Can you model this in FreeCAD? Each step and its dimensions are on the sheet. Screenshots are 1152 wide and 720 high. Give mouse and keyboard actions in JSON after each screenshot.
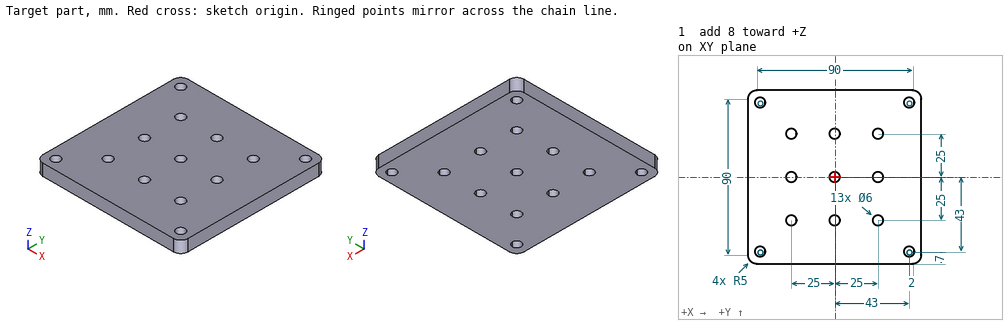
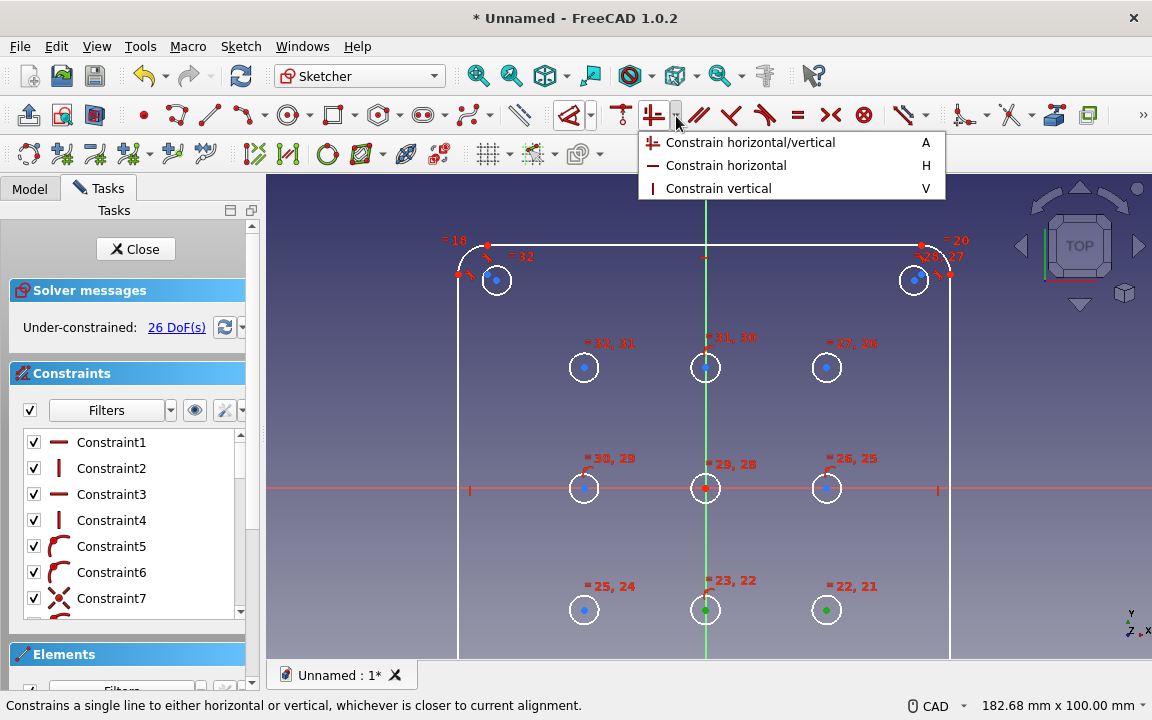
{"action": "left_click", "coordinate": [792, 166]}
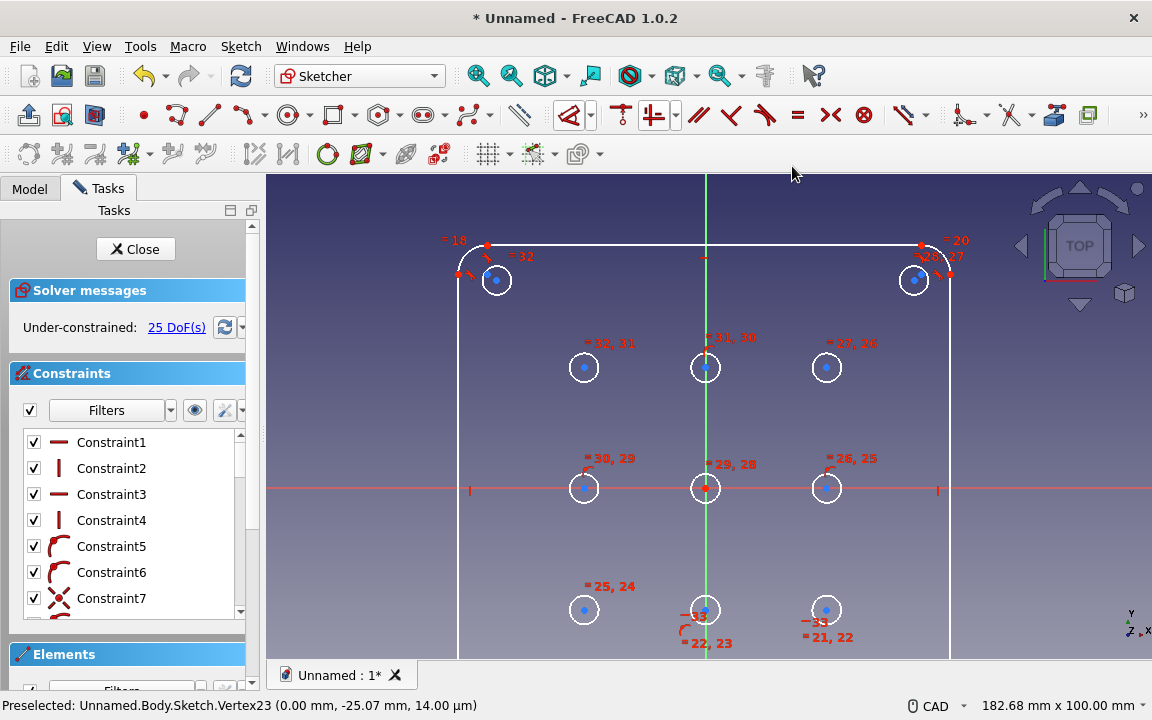
{"action": "scroll", "coordinate": [706, 610], "scroll_direction": "up", "scroll_amount": 4}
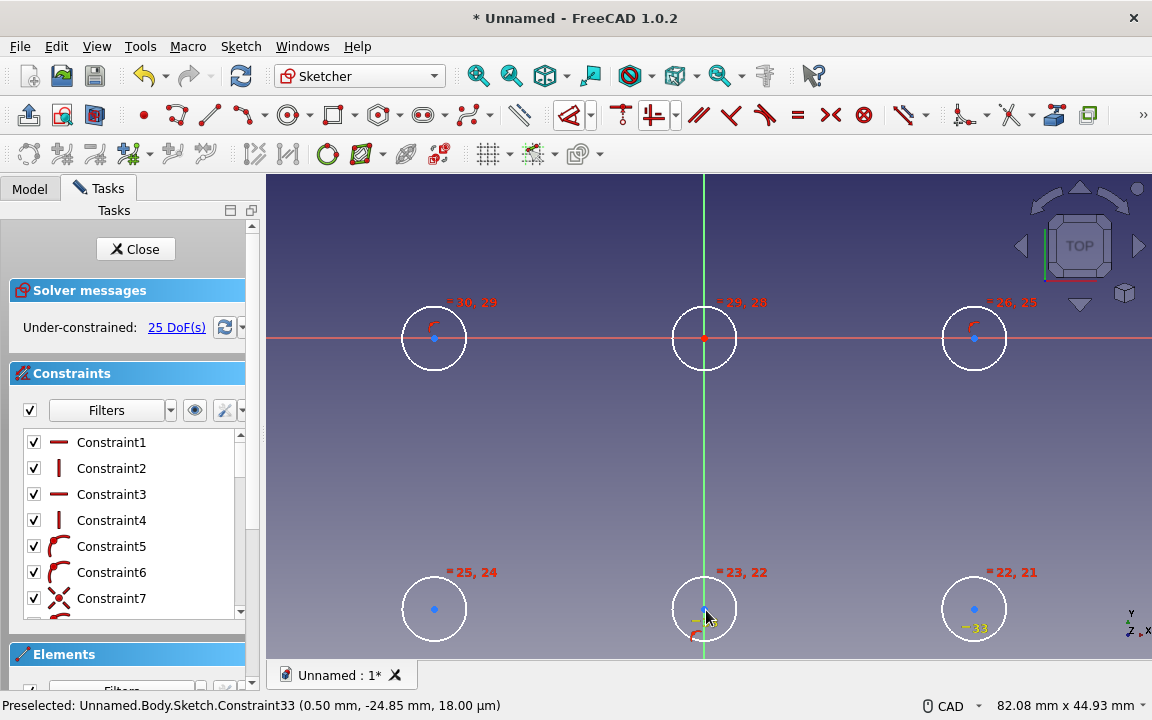
{"action": "left_click", "coordinate": [704, 609]}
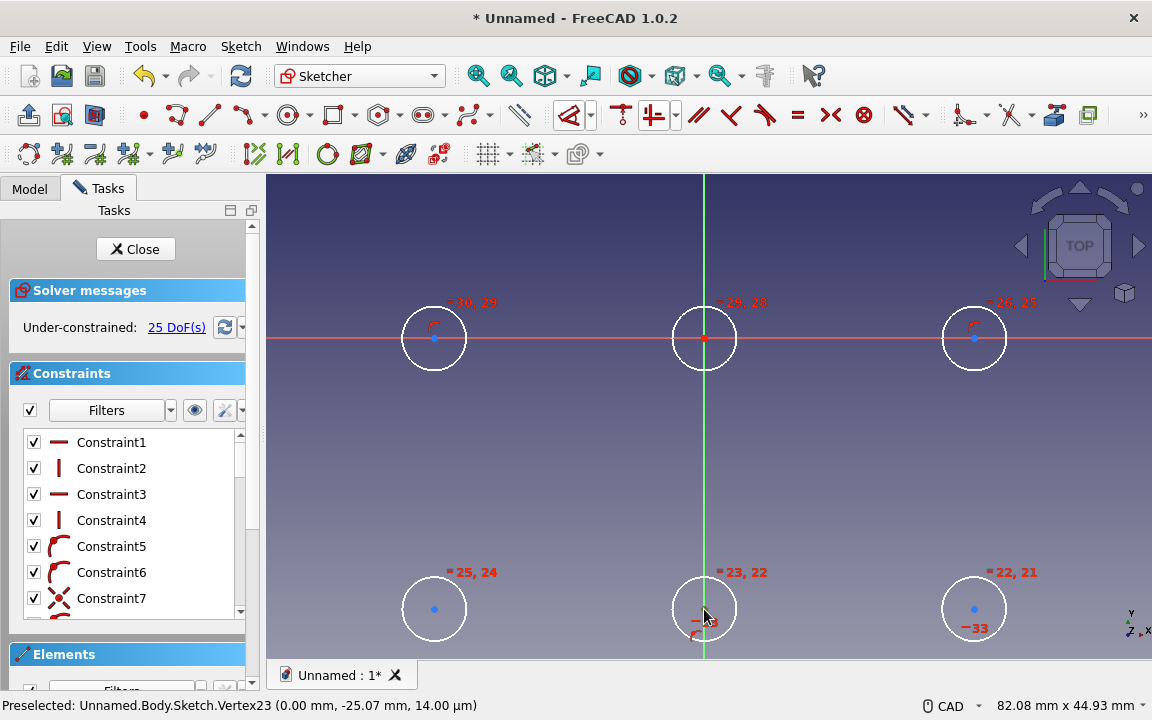
{"action": "left_click", "coordinate": [434, 609]}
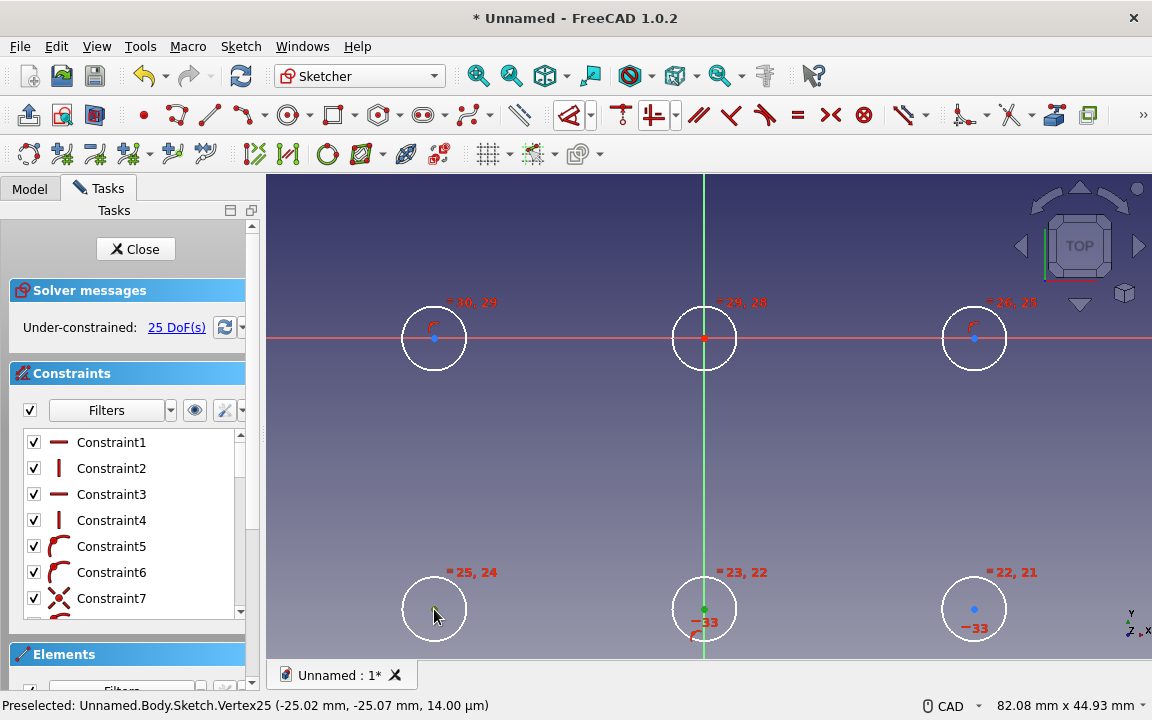
{"action": "key", "text": "h"}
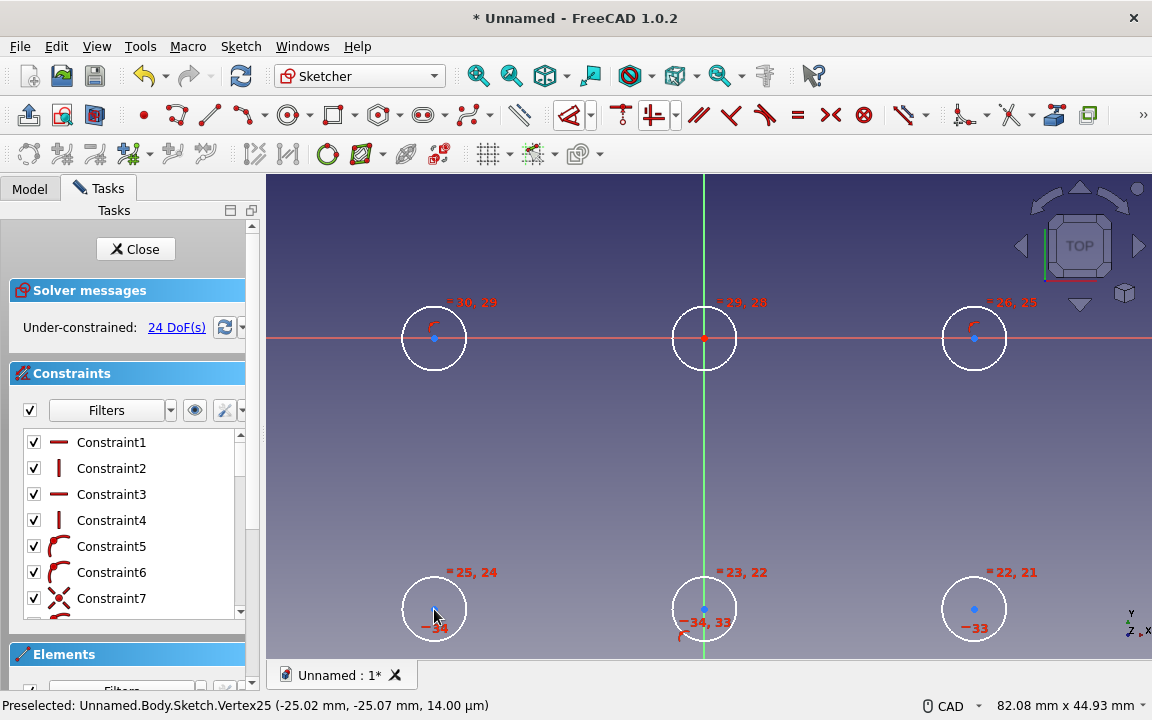
{"action": "left_click", "coordinate": [974, 609]}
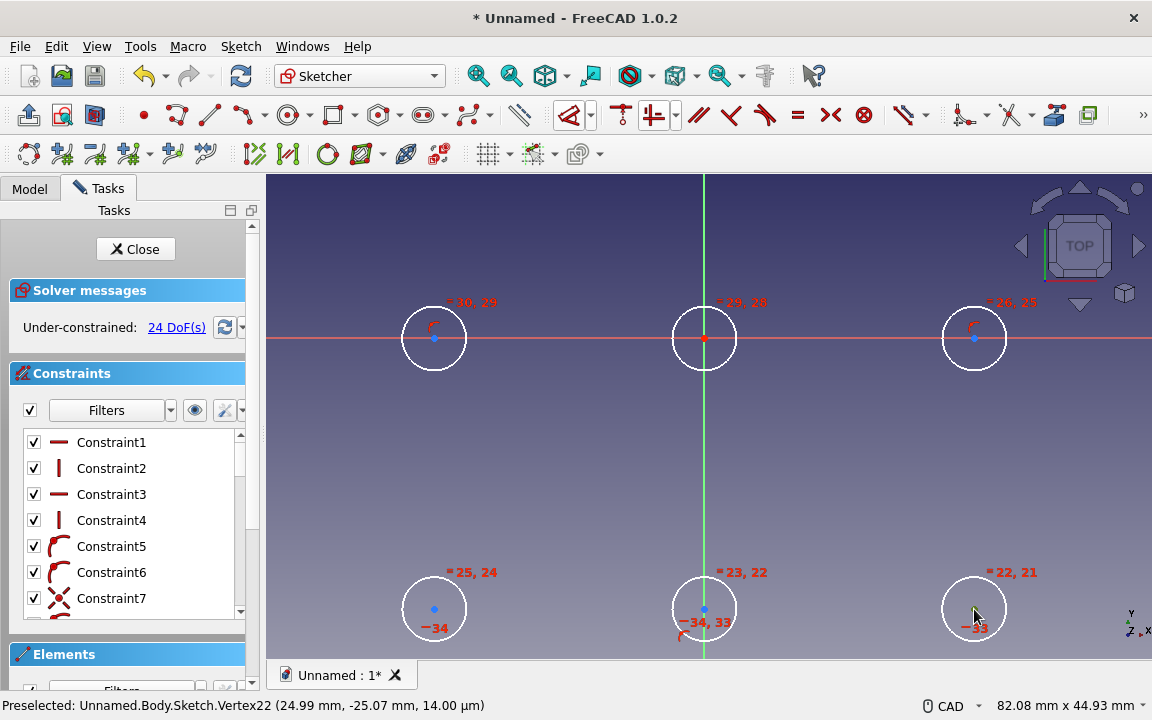
{"action": "left_click", "coordinate": [974, 338]}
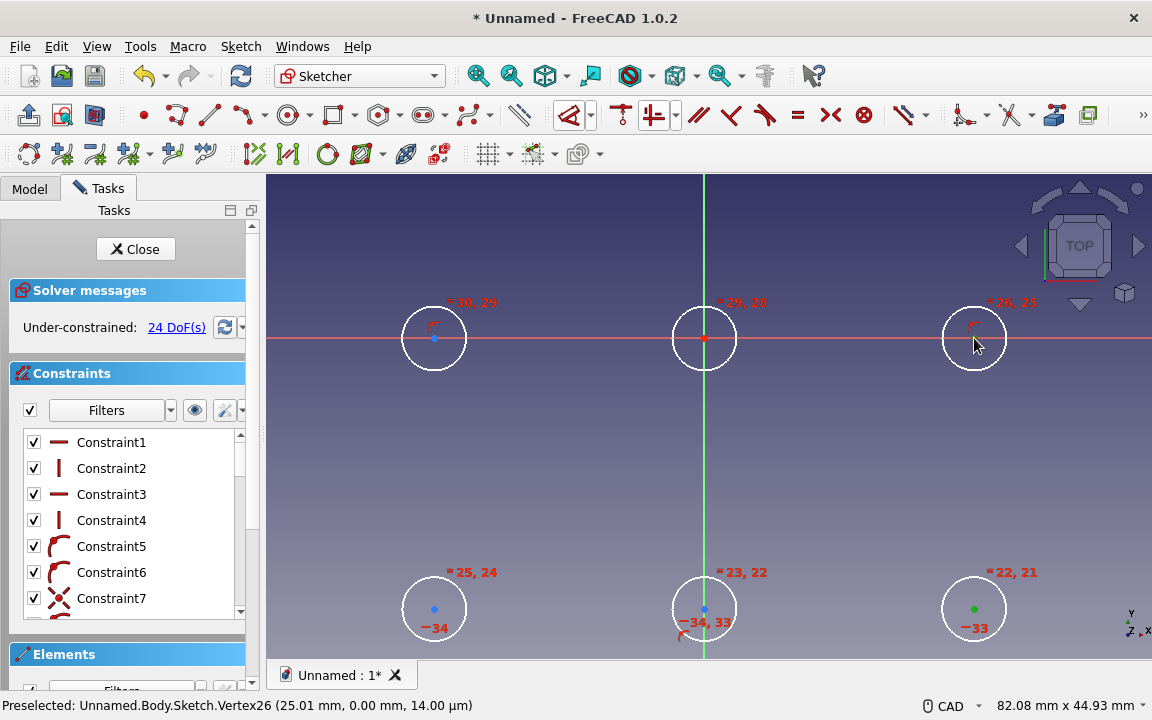
{"action": "key", "text": "v"}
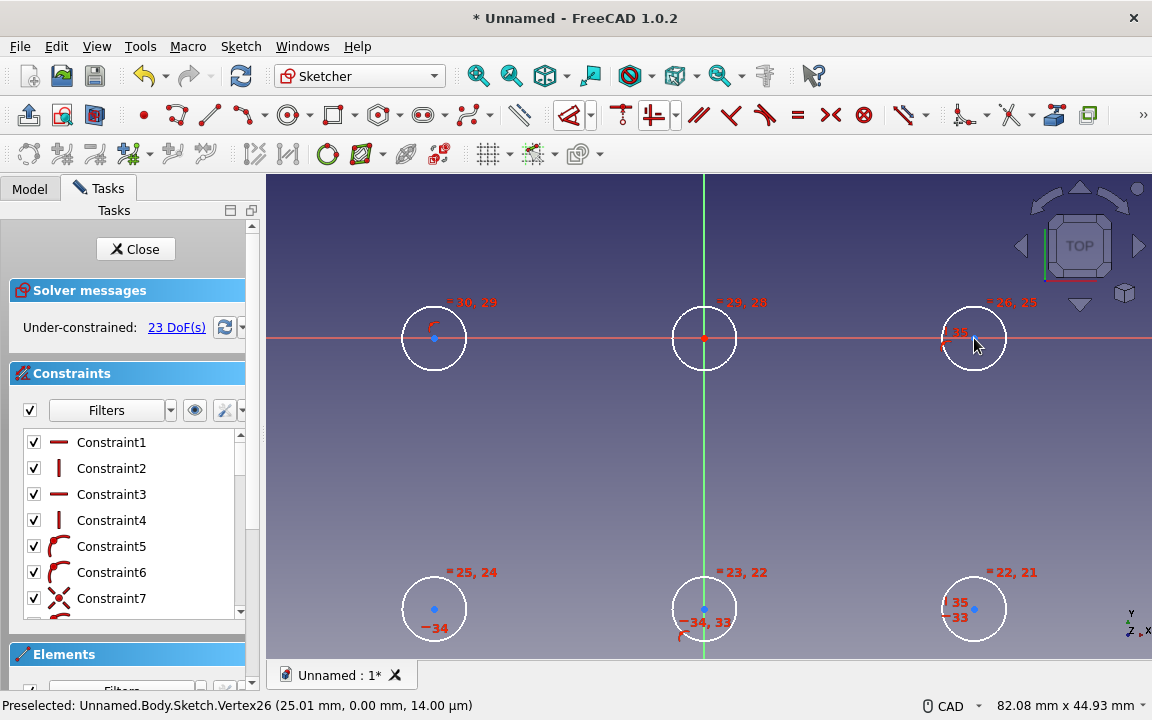
{"action": "left_click", "coordinate": [974, 338]}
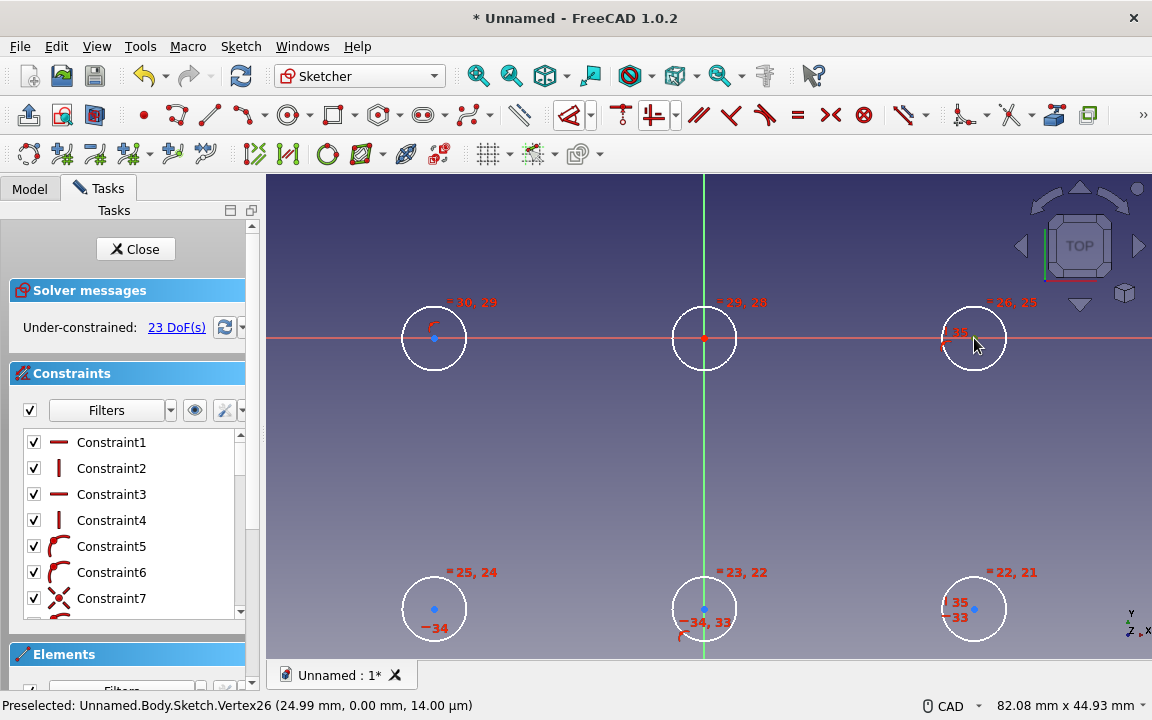
{"action": "scroll", "coordinate": [613, 450], "scroll_direction": "down", "scroll_amount": 6}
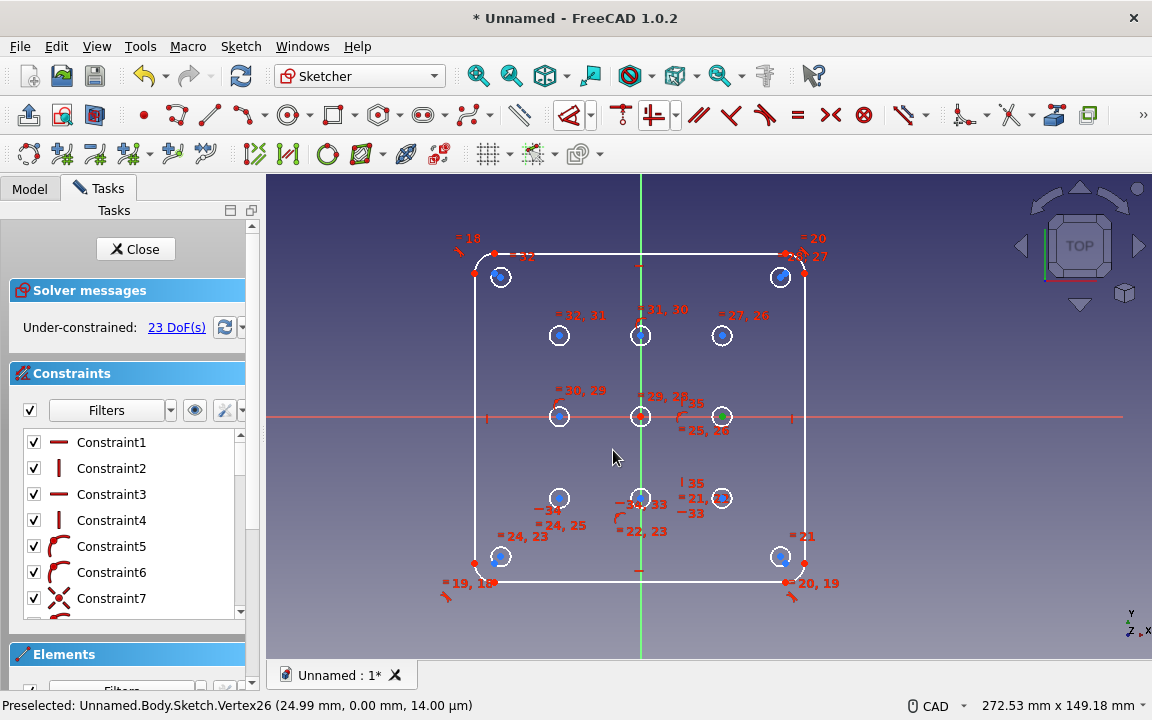
{"action": "left_click", "coordinate": [722, 336]}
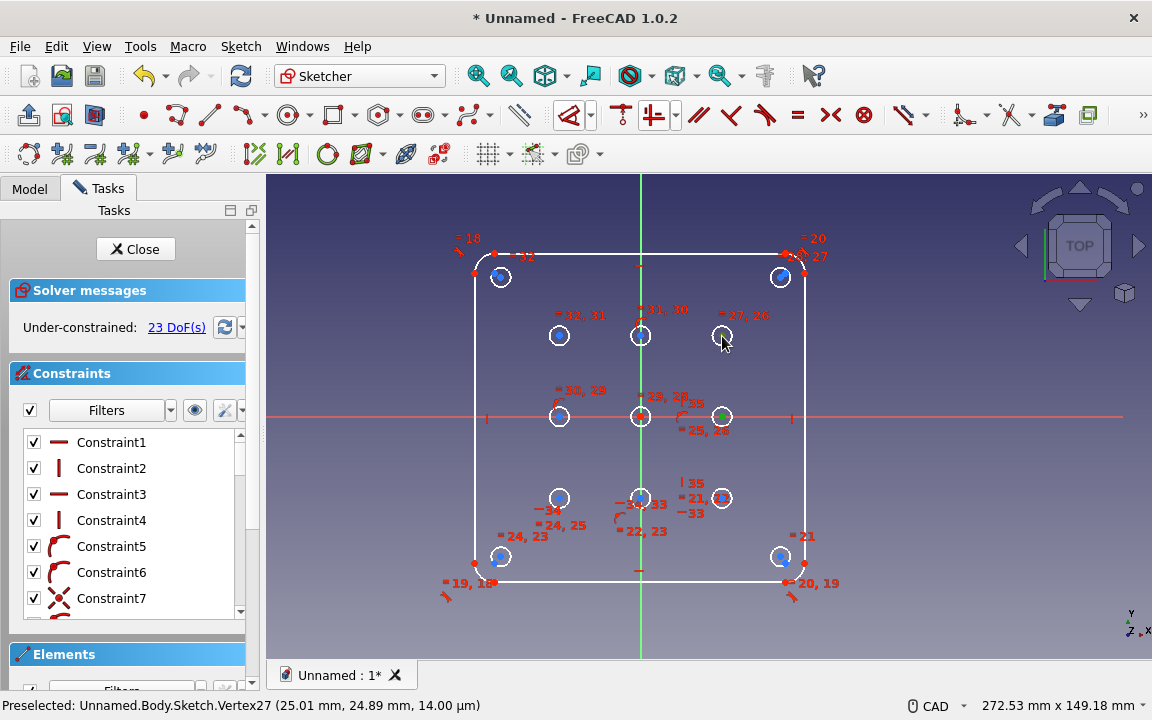
{"action": "key", "text": "v"}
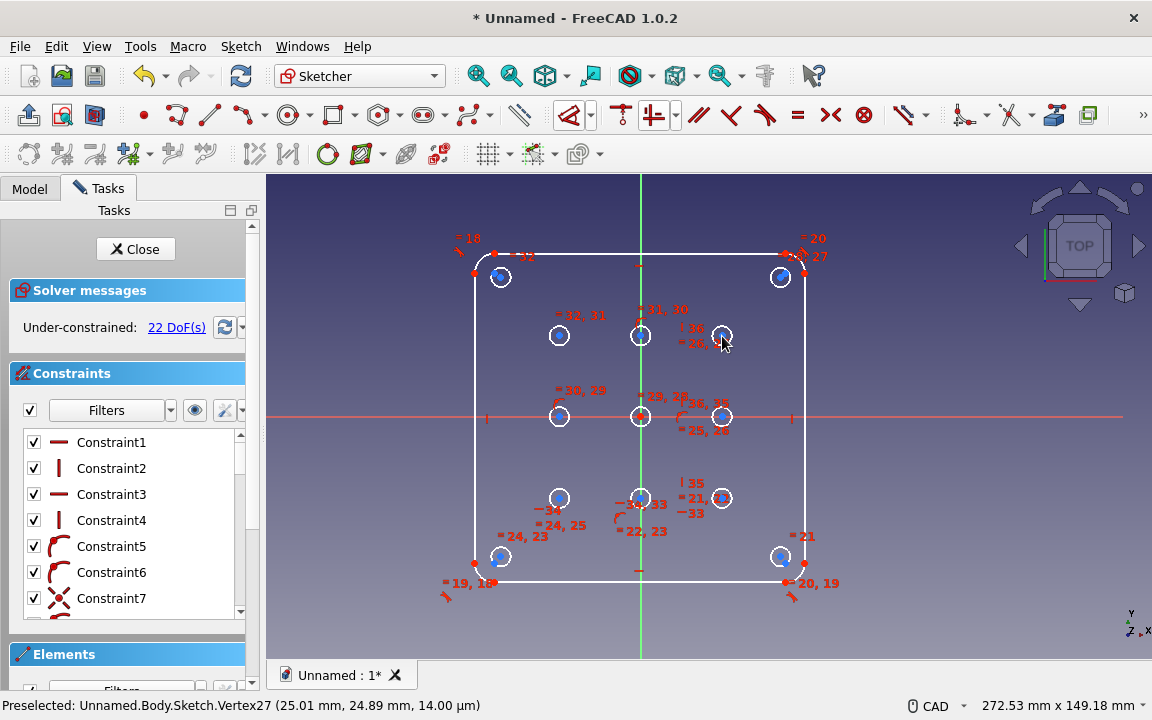
{"action": "left_click", "coordinate": [559, 498]}